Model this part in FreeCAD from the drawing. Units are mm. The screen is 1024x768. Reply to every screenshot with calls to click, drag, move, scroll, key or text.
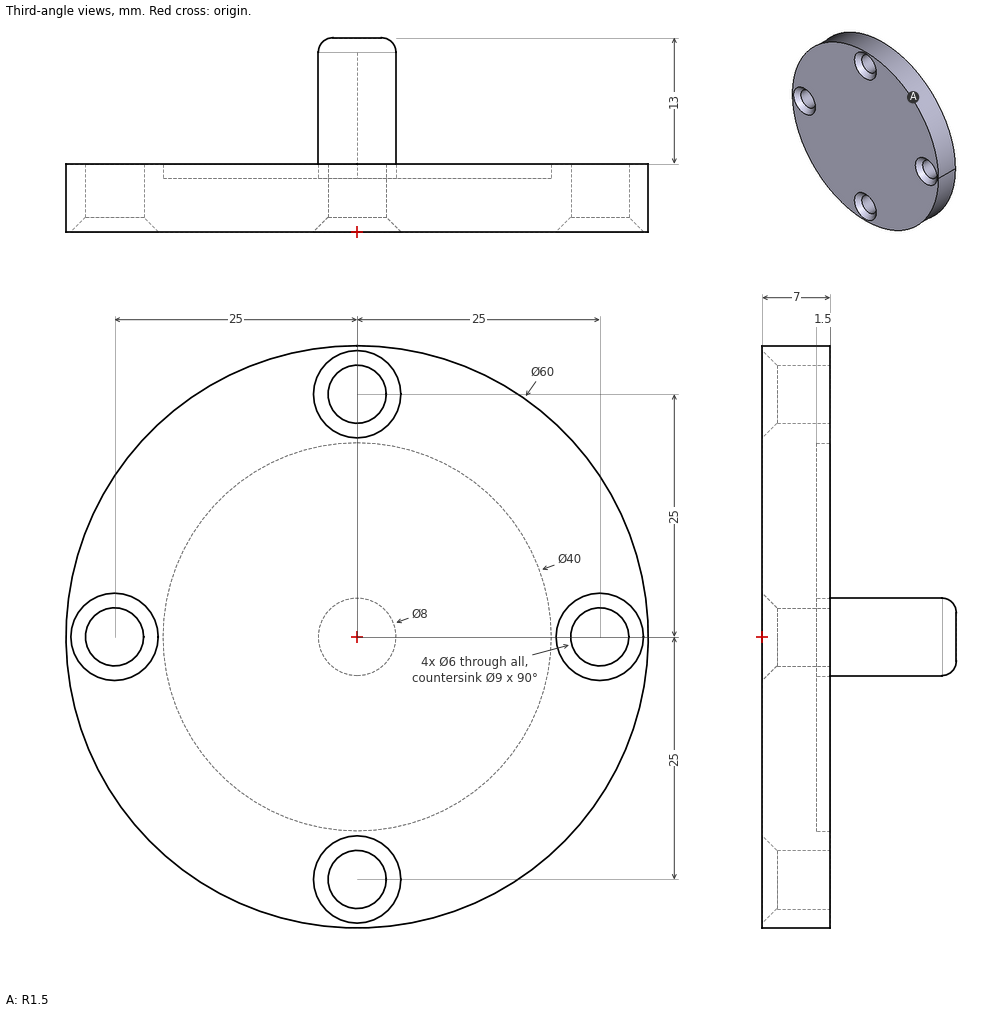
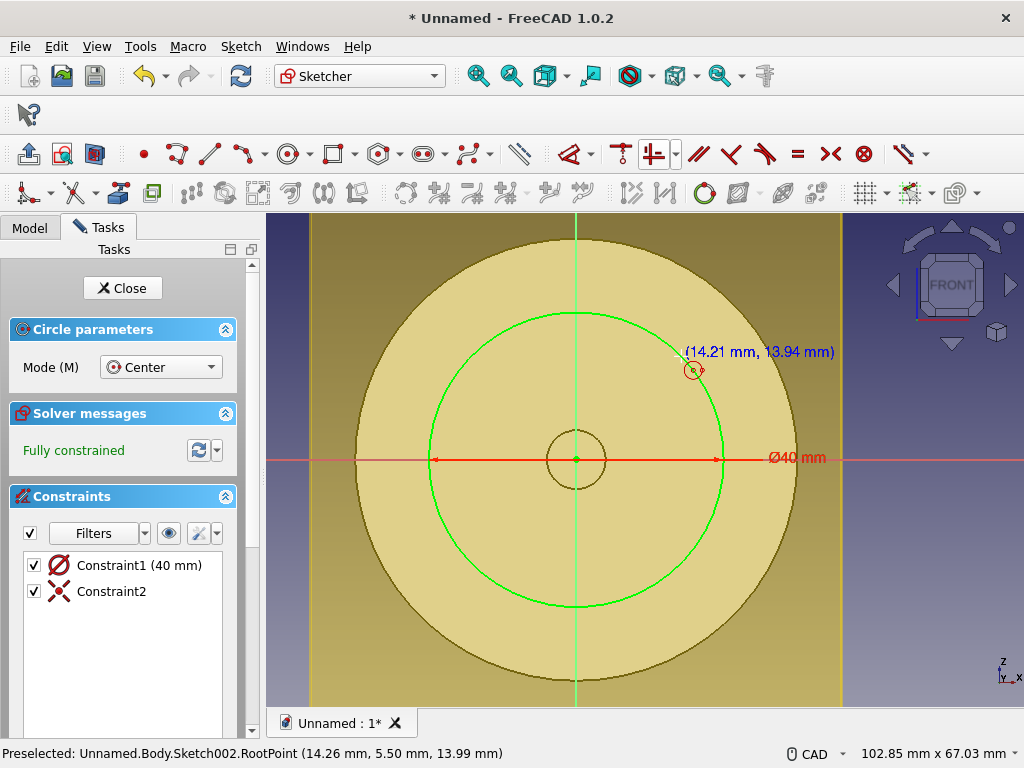
click(576, 460)
move(597, 439)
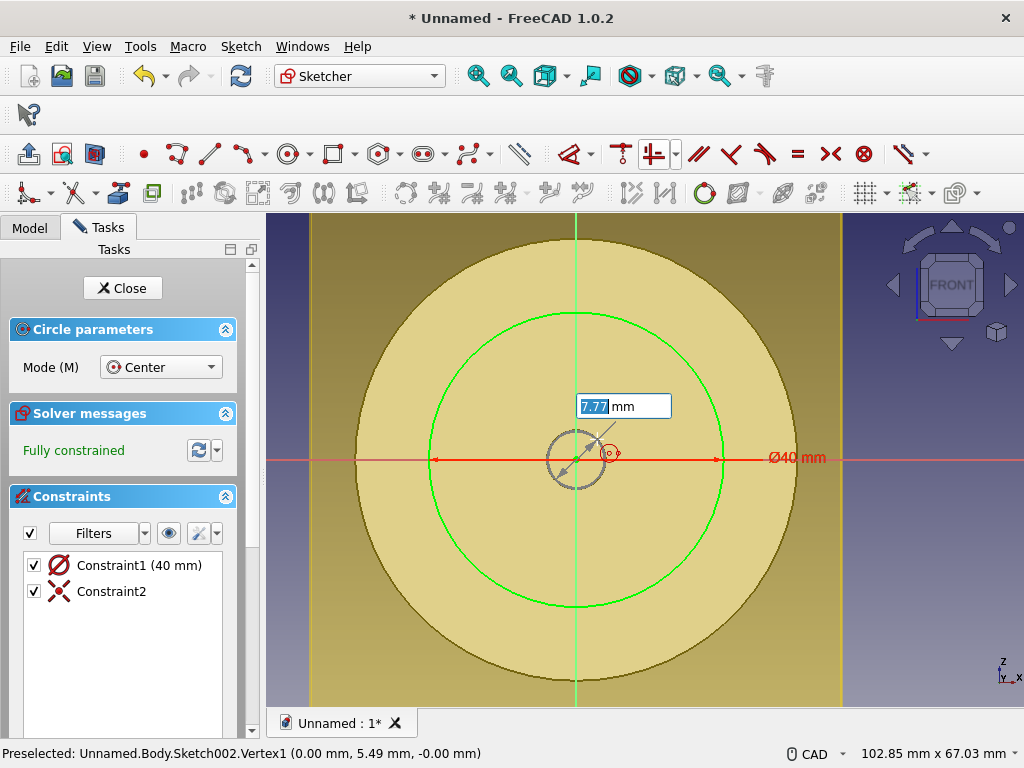
text(8)
key(Return)
key(Escape)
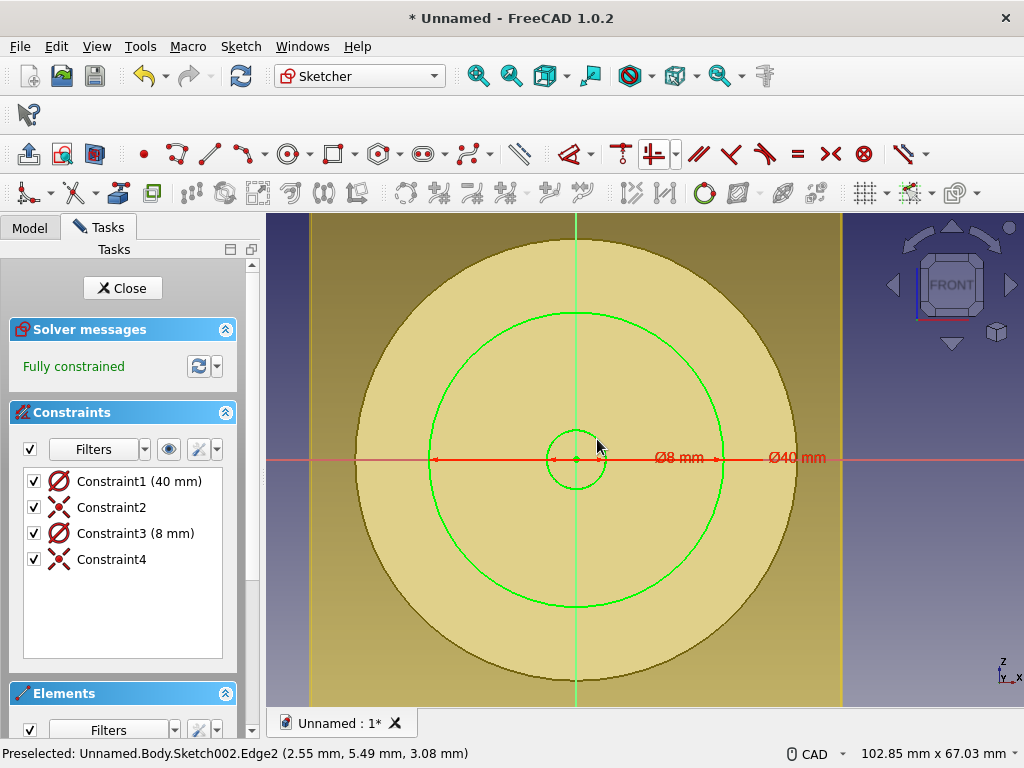
click(123, 288)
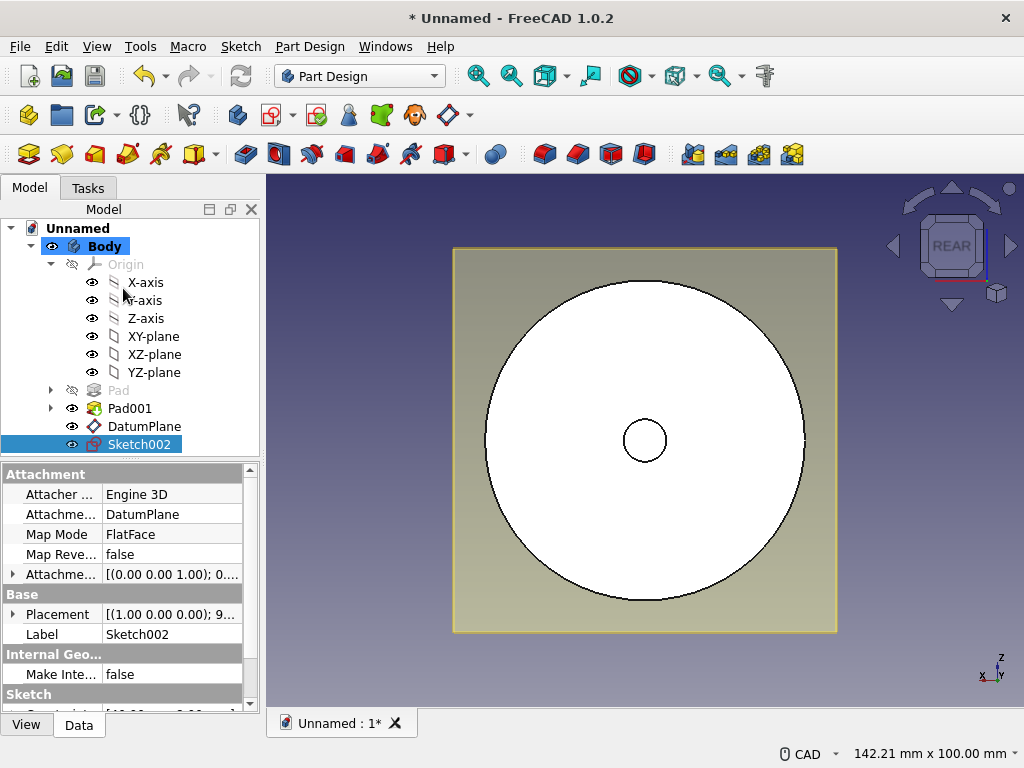
click(246, 154)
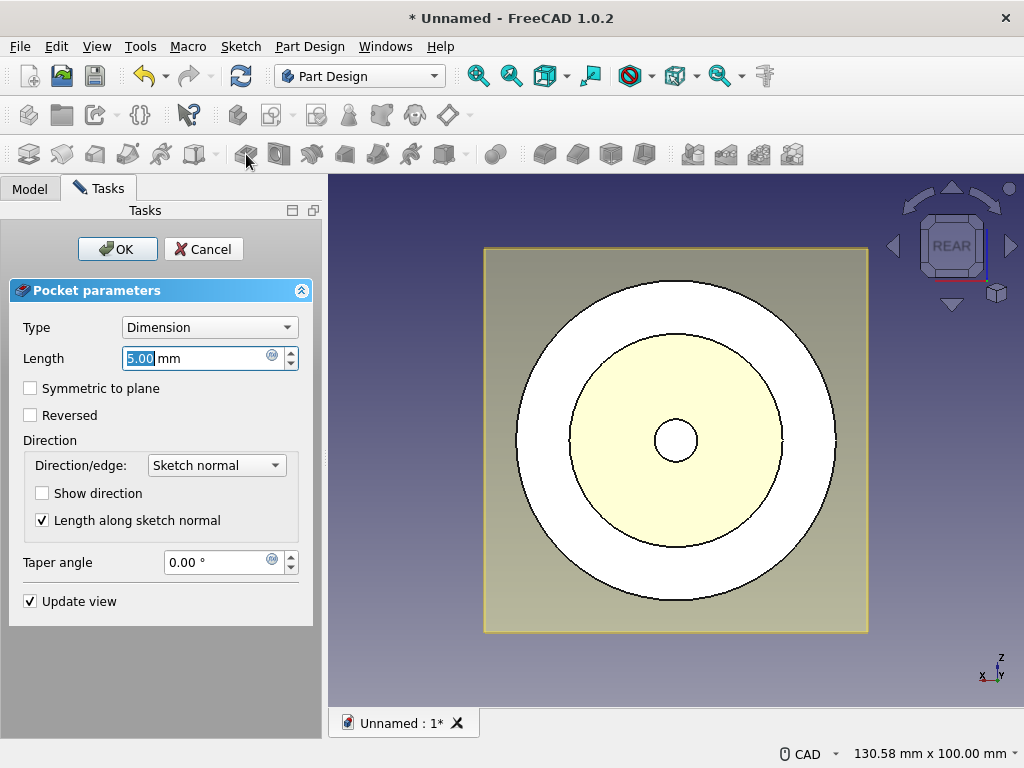
text(1.5)
key(Tab)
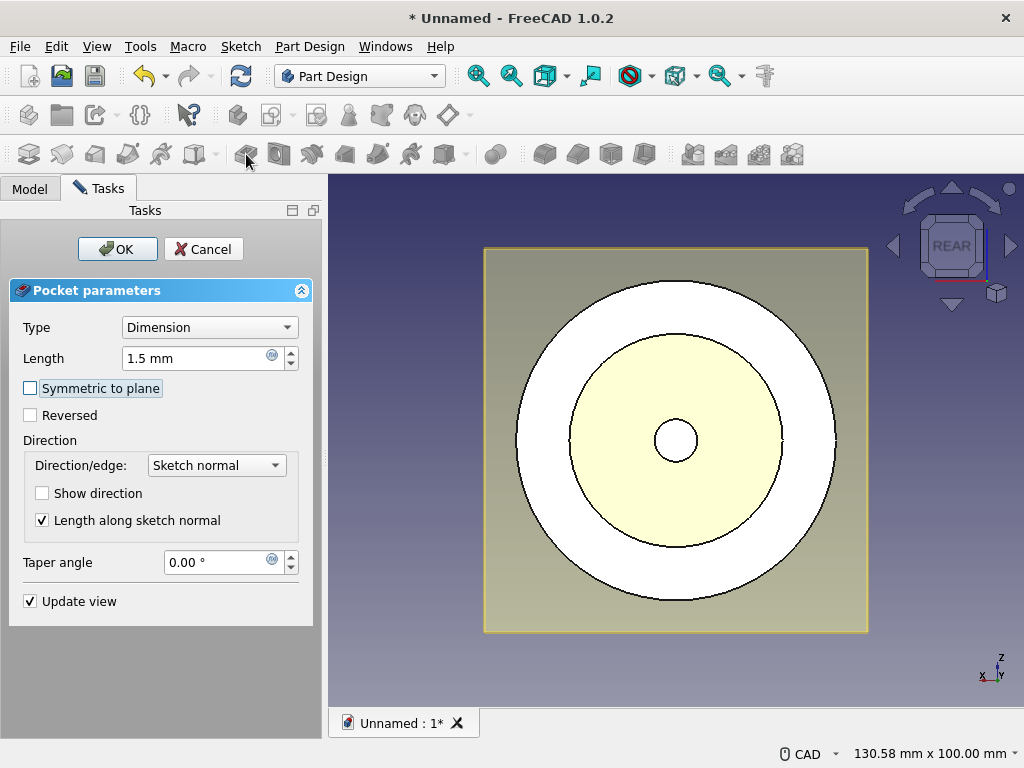
click(118, 249)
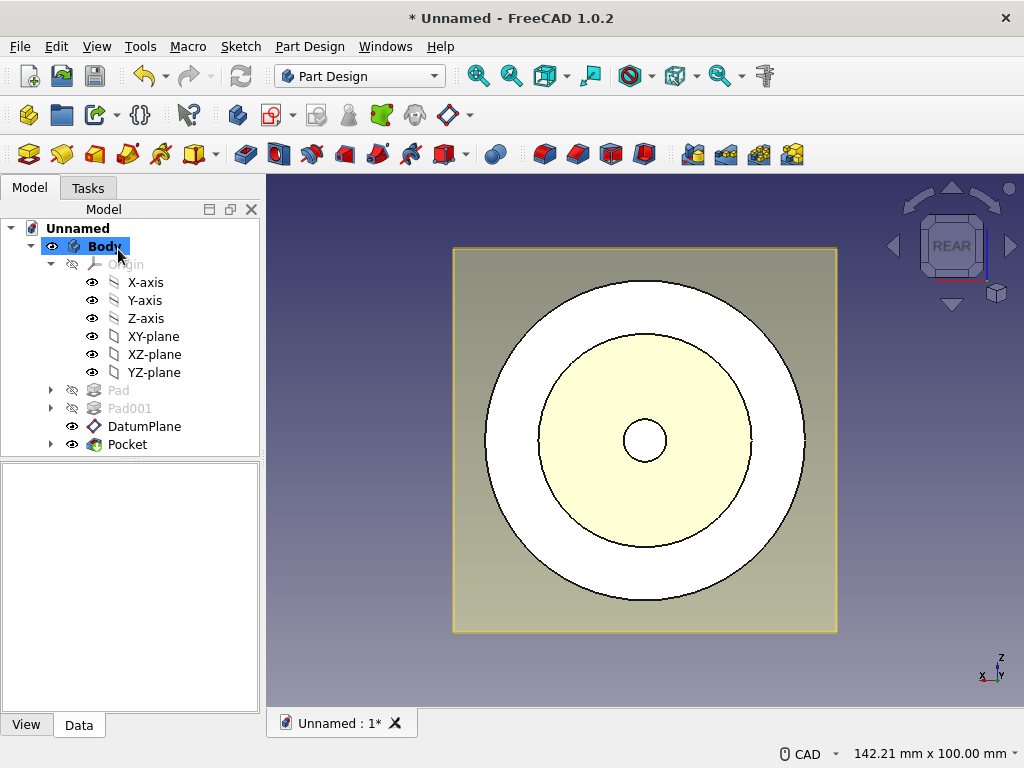
click(117, 426)
key(space)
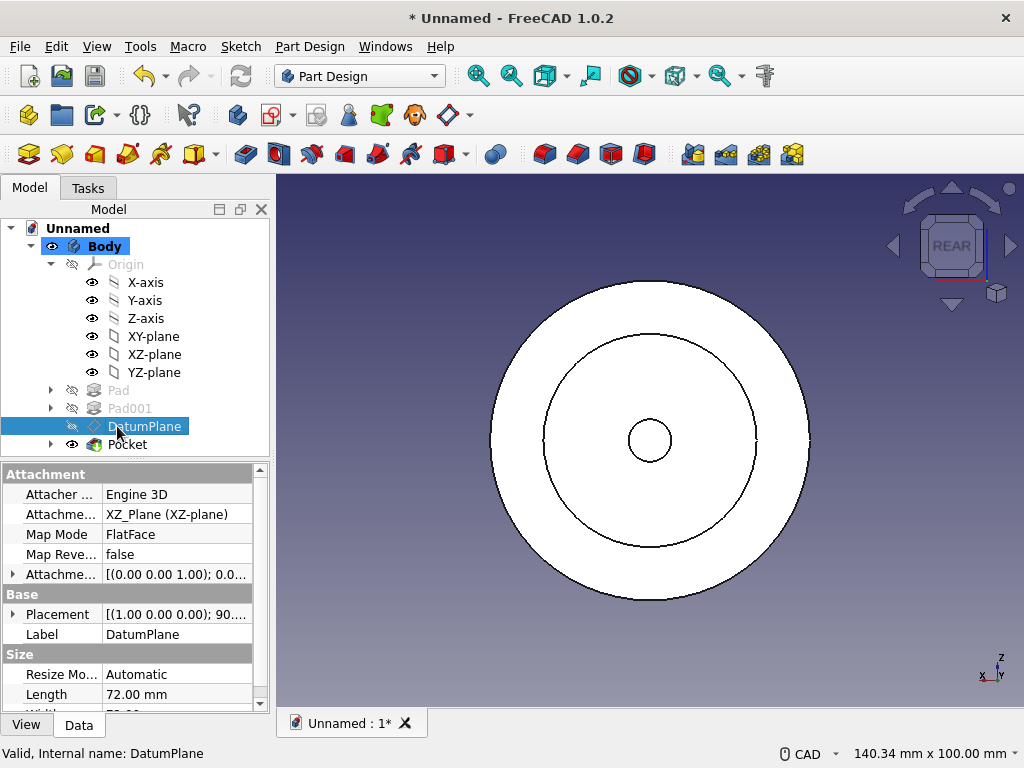
click(316, 667)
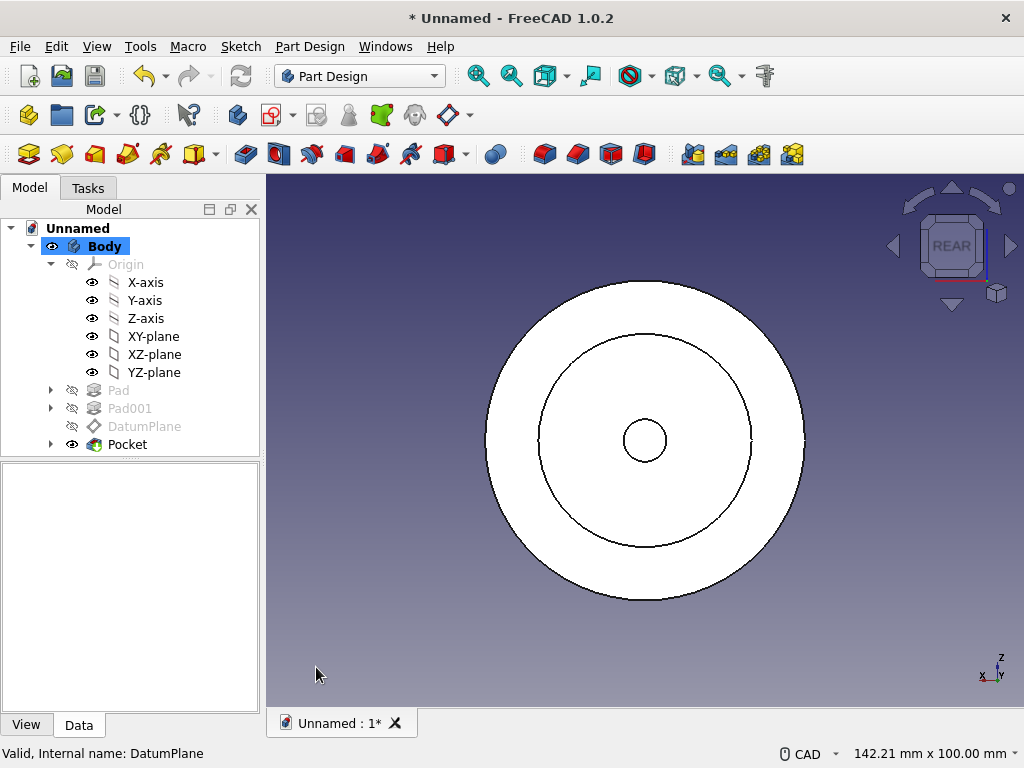
click(270, 116)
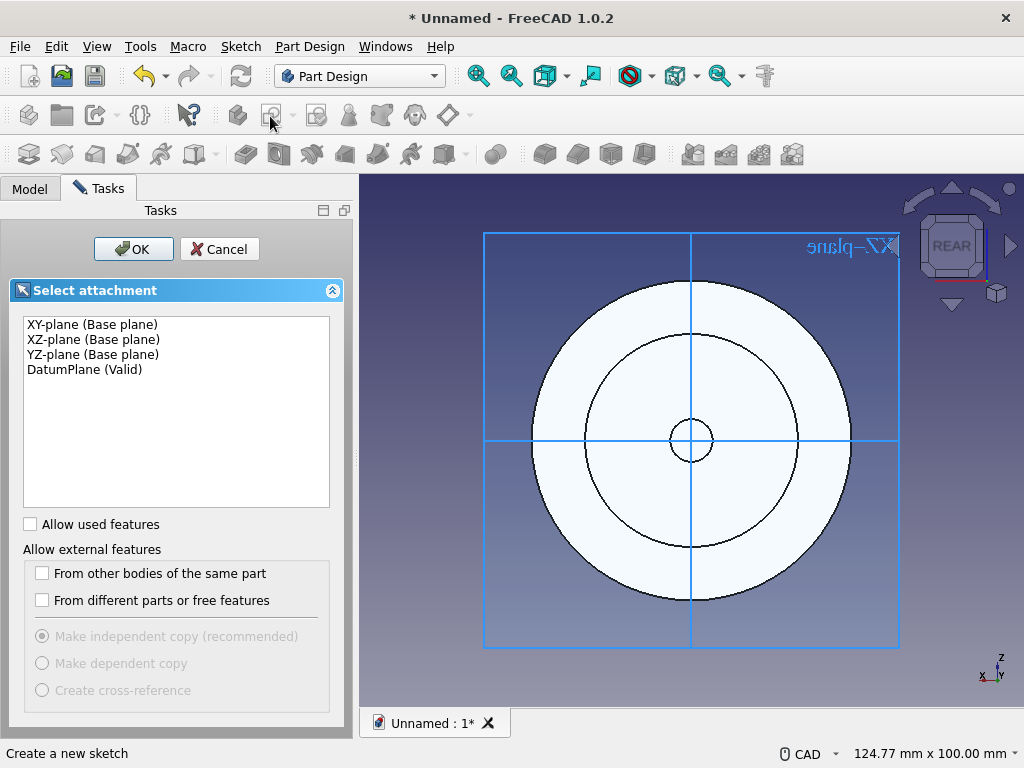
click(84, 340)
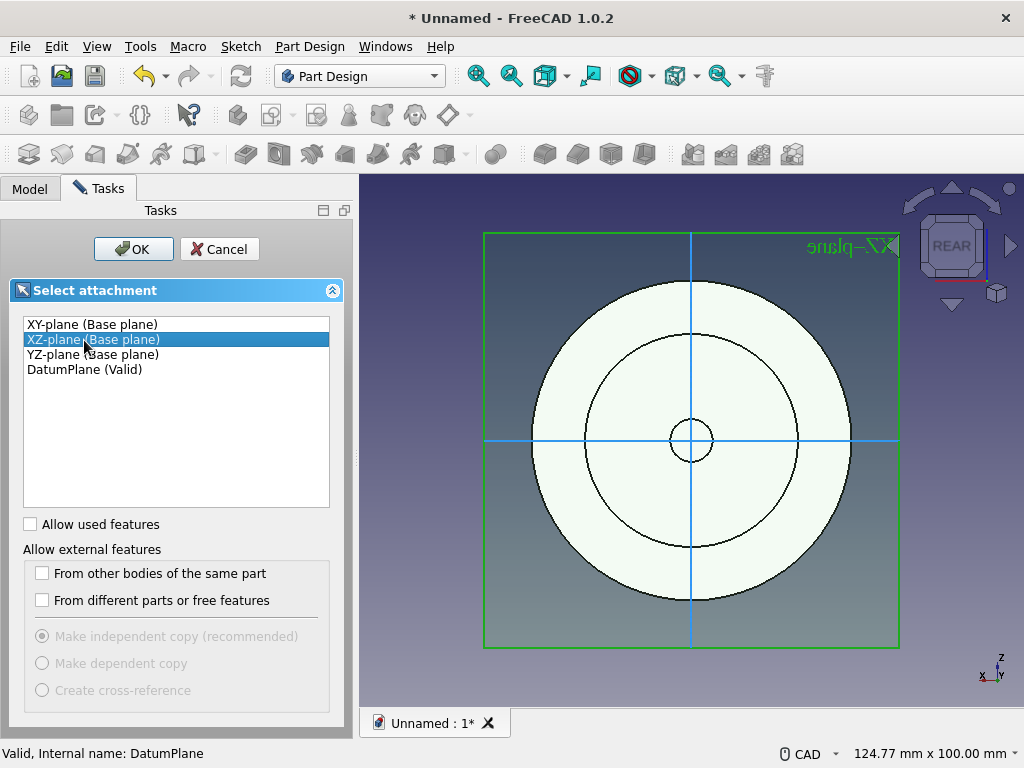
click(134, 249)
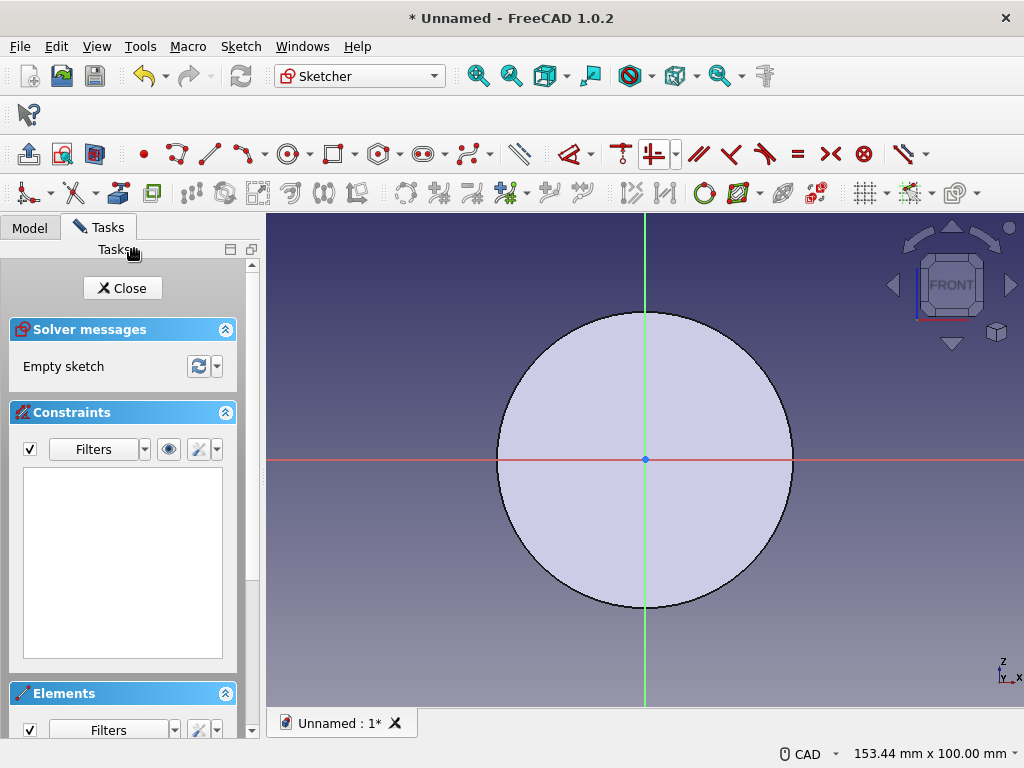
click(288, 154)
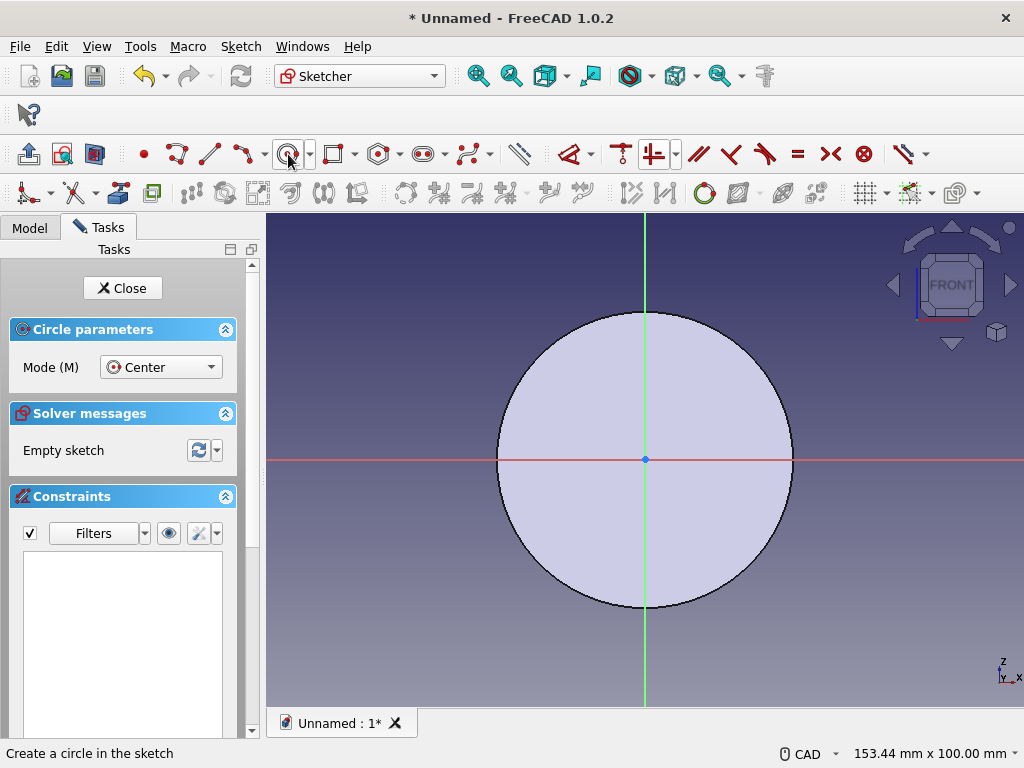
scroll(768, 460, up, 3)